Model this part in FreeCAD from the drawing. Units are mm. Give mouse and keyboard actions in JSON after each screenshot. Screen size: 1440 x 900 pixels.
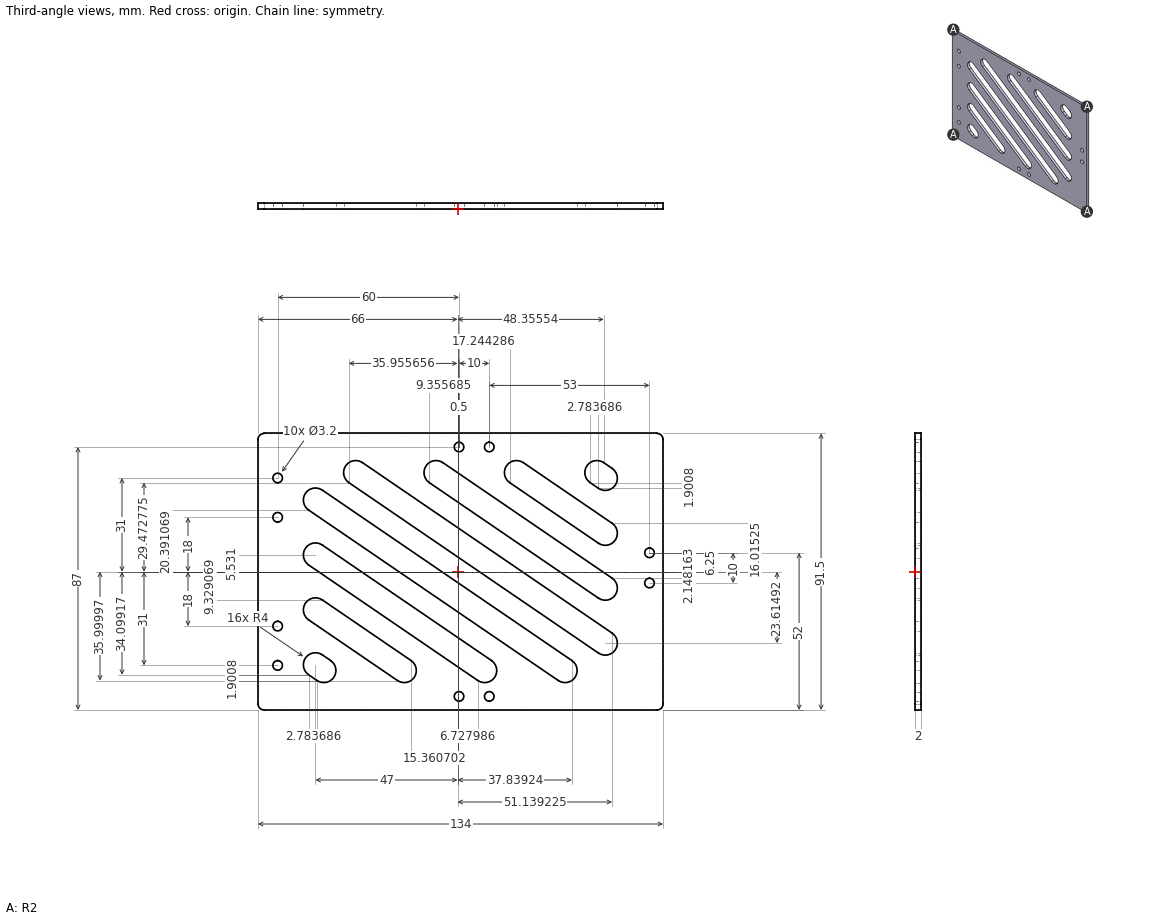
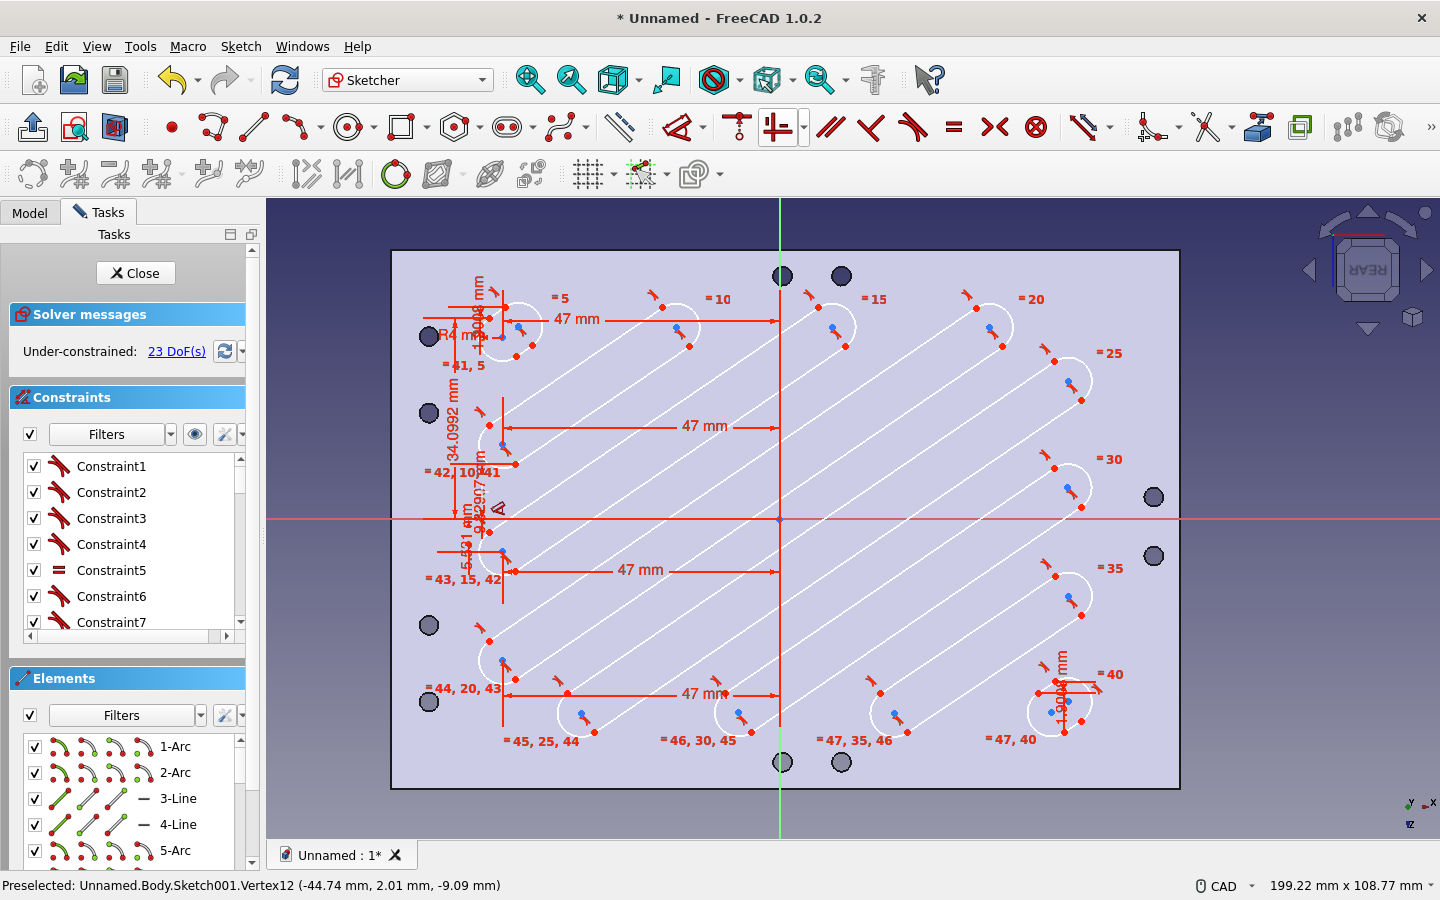
{"action": "left_click", "coordinate": [663, 308]}
{"action": "left_click", "coordinate": [629, 413]}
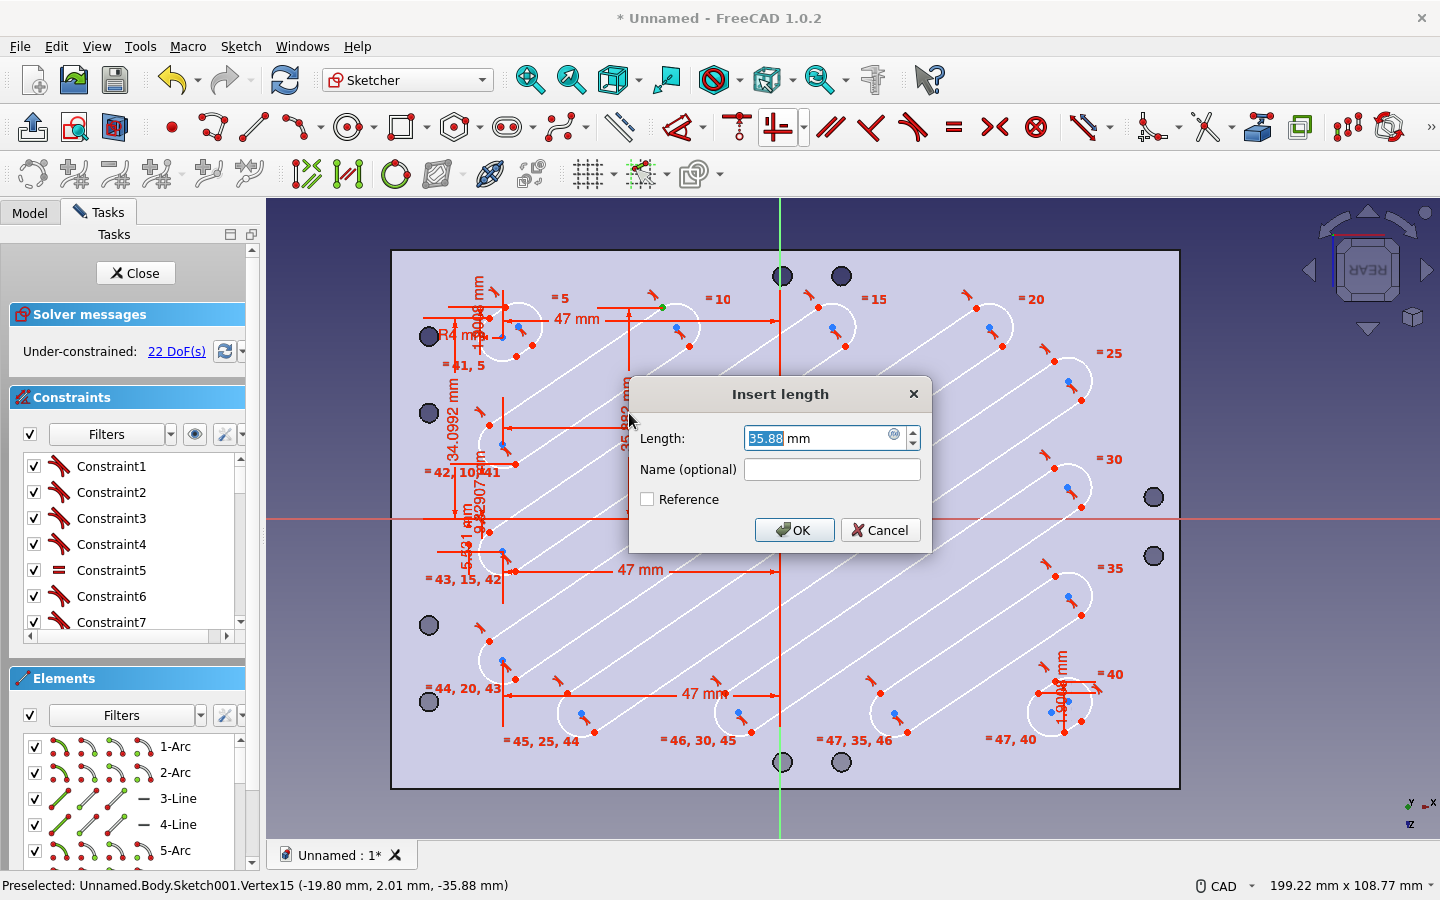
{"action": "type", "text": "35.99997"}
{"action": "key", "text": "Return"}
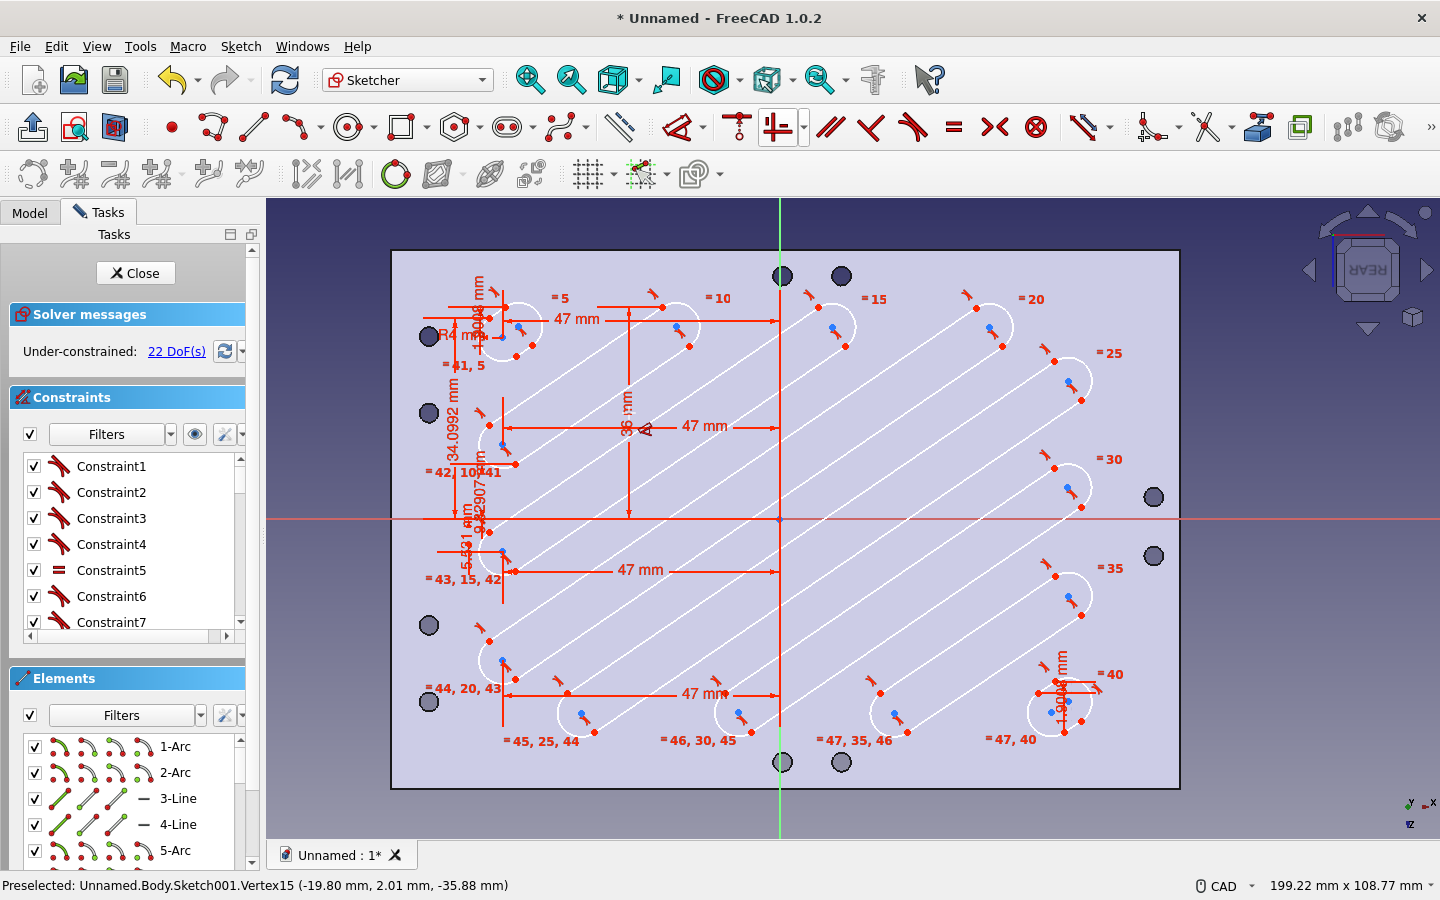
{"action": "left_click", "coordinate": [819, 308]}
{"action": "left_click", "coordinate": [799, 274]}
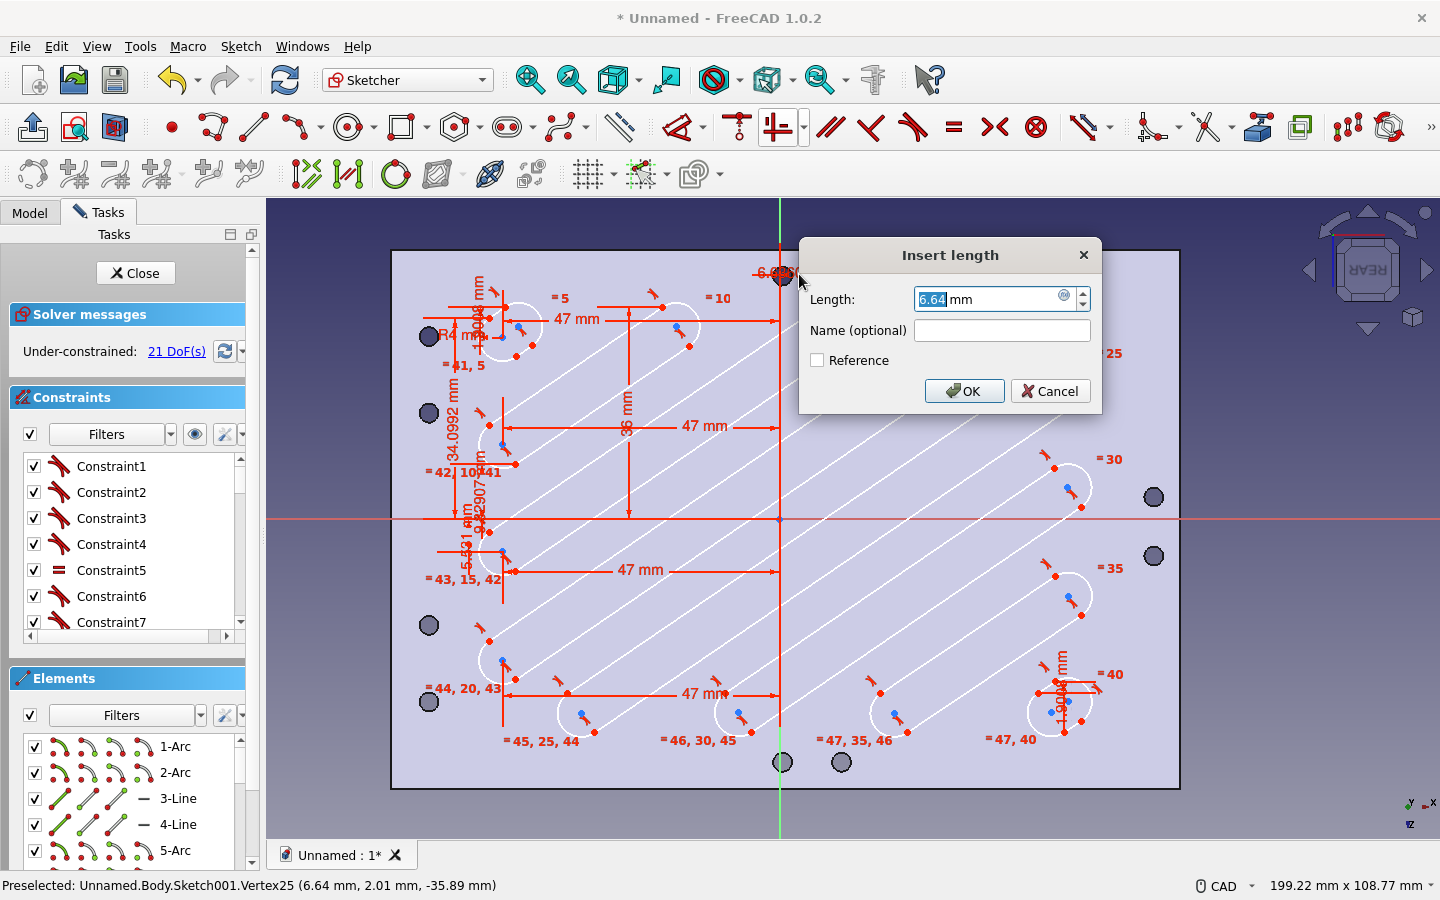
{"action": "type", "text": "6.727986"}
{"action": "key", "text": "Return"}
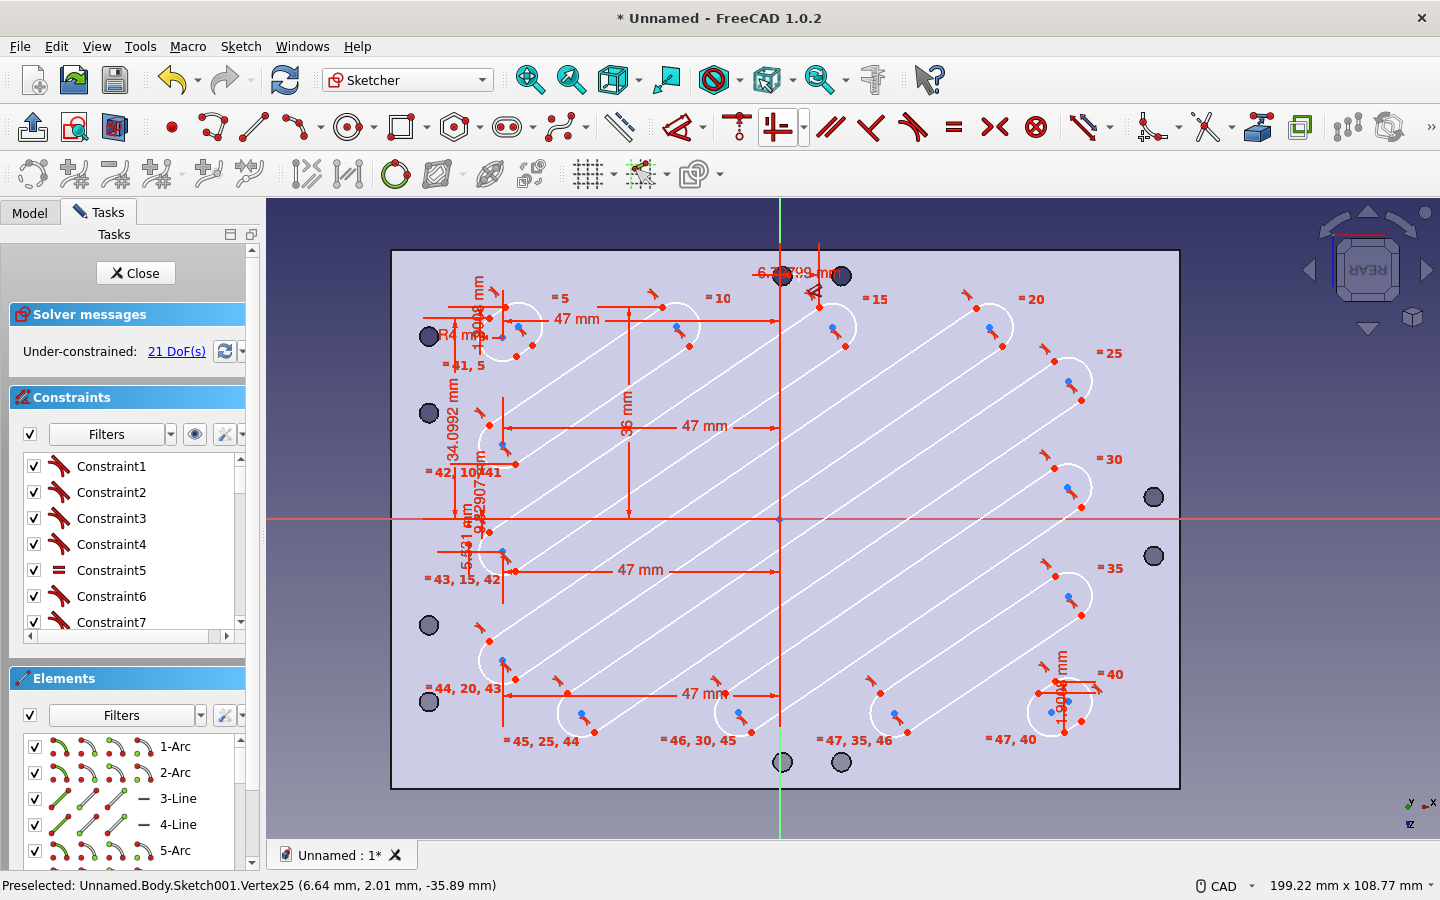
{"action": "left_click", "coordinate": [819, 308]}
{"action": "left_click", "coordinate": [853, 413]}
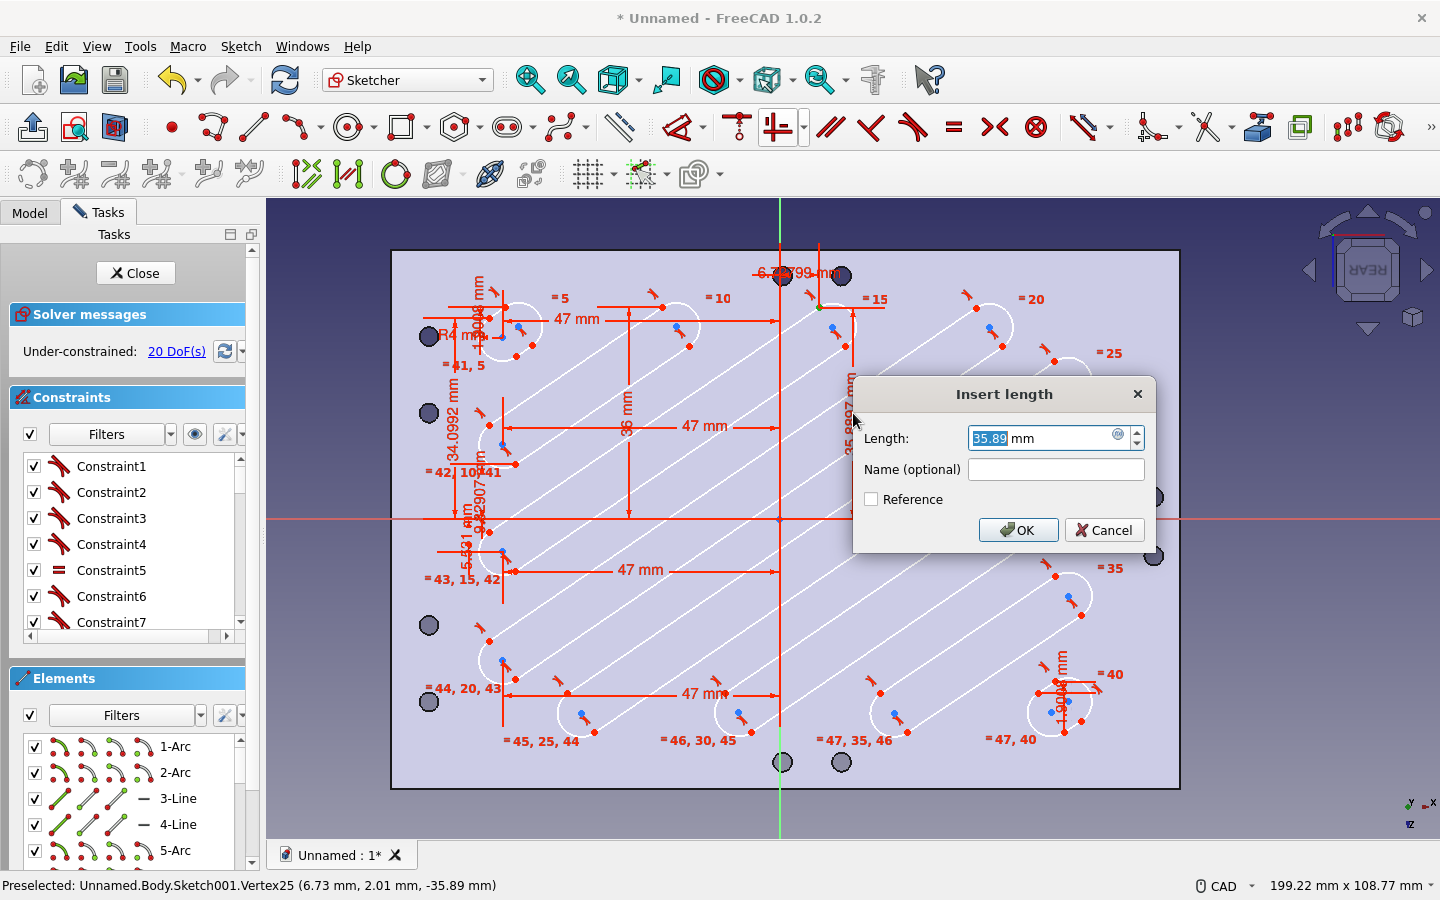
{"action": "type", "text": "35.99997"}
{"action": "key", "text": "Return"}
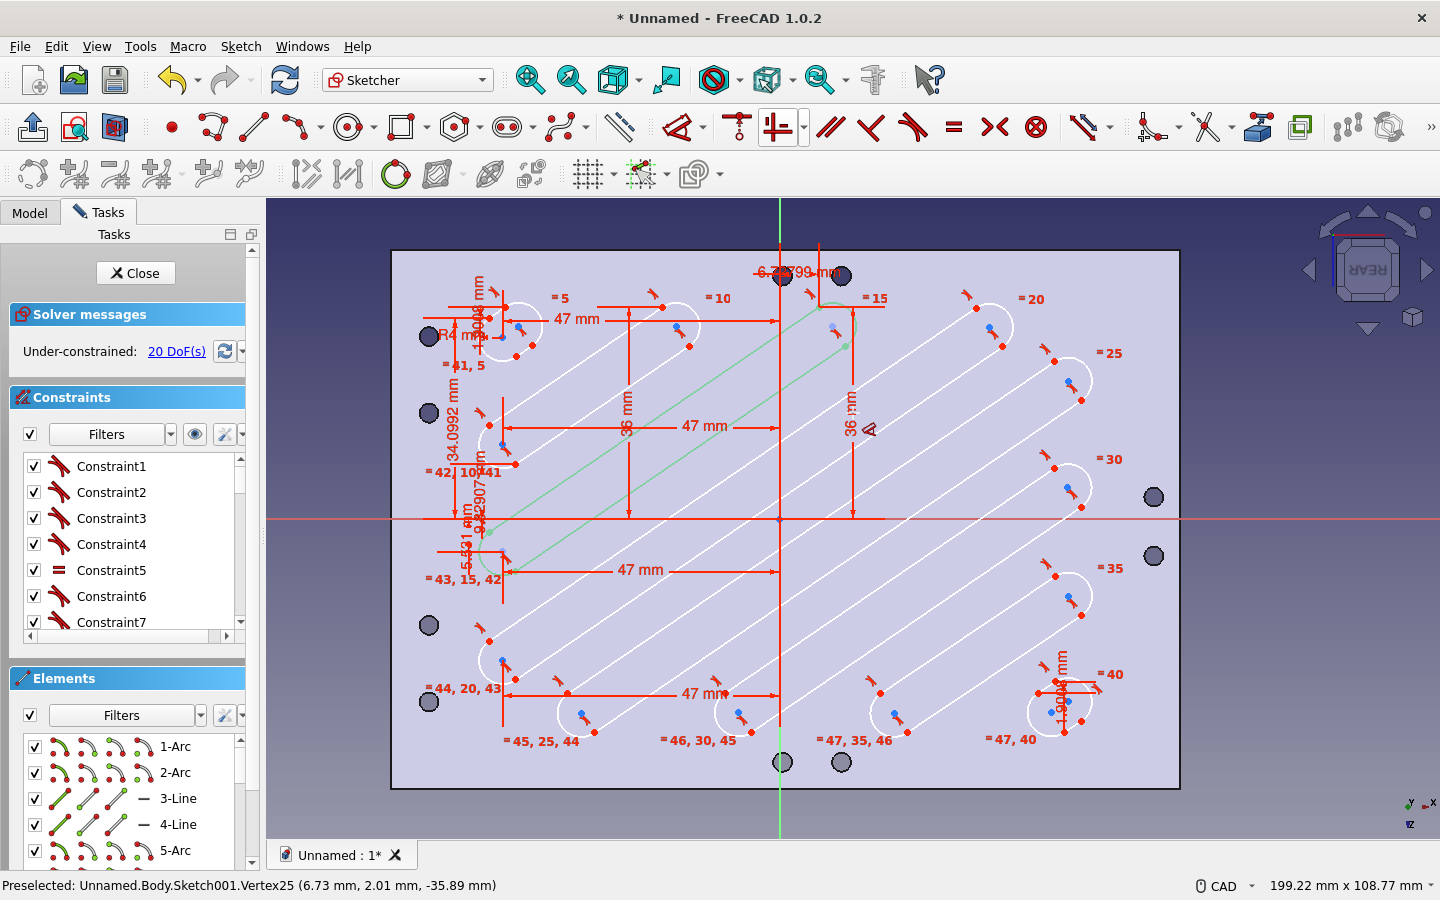
{"action": "left_click", "coordinate": [1003, 347]}
{"action": "left_click", "coordinate": [891, 313]}